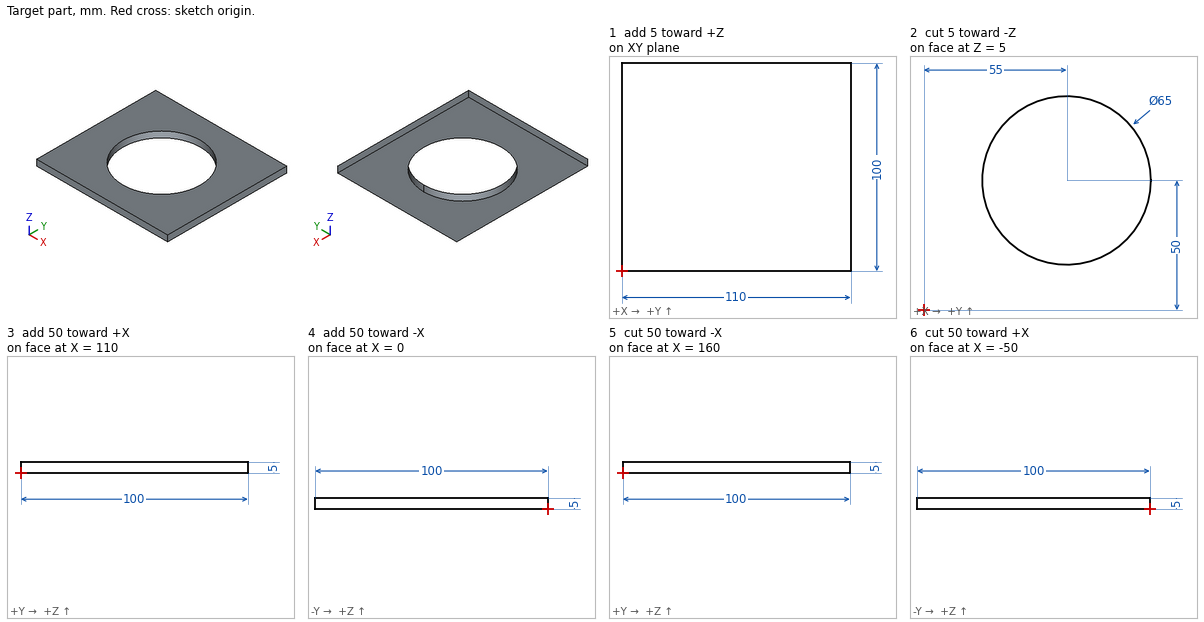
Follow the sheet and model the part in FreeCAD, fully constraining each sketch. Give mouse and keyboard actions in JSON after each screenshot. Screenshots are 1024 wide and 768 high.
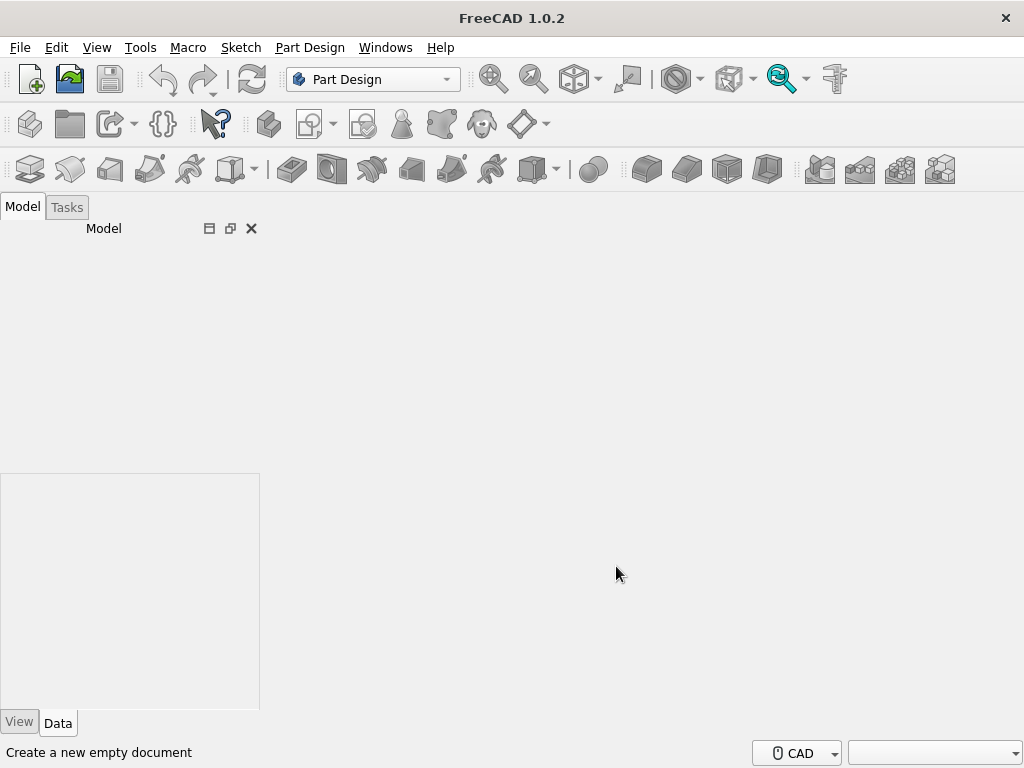
{"action": "left_click", "coordinate": [30, 80]}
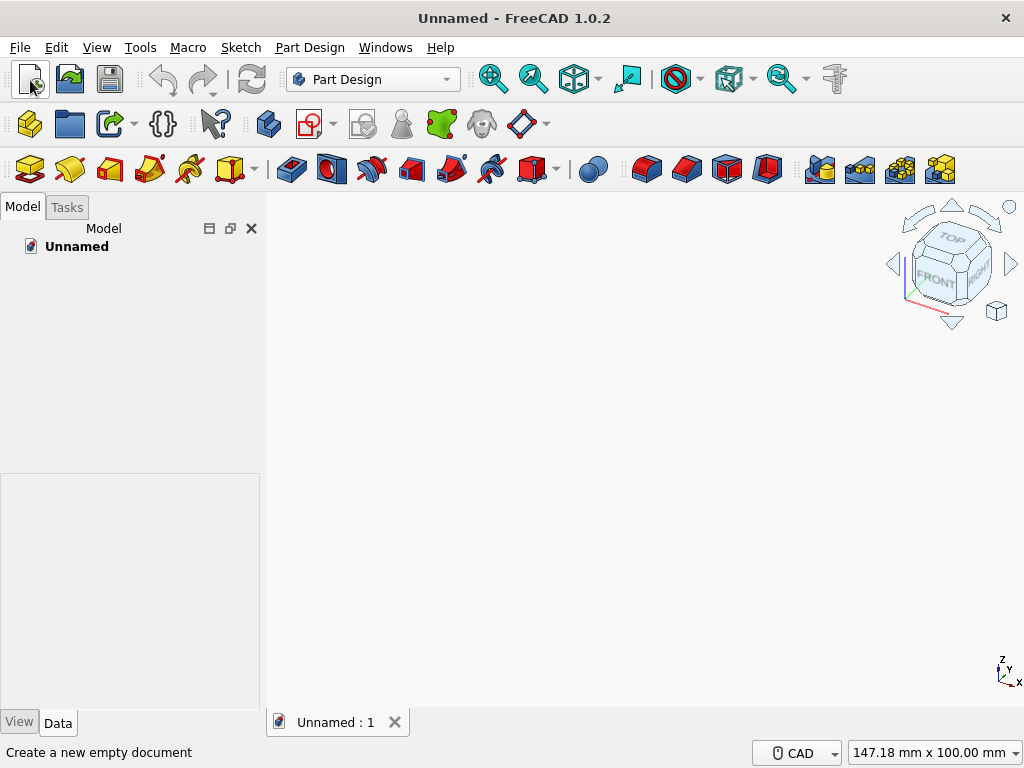
{"action": "left_click", "coordinate": [310, 124]}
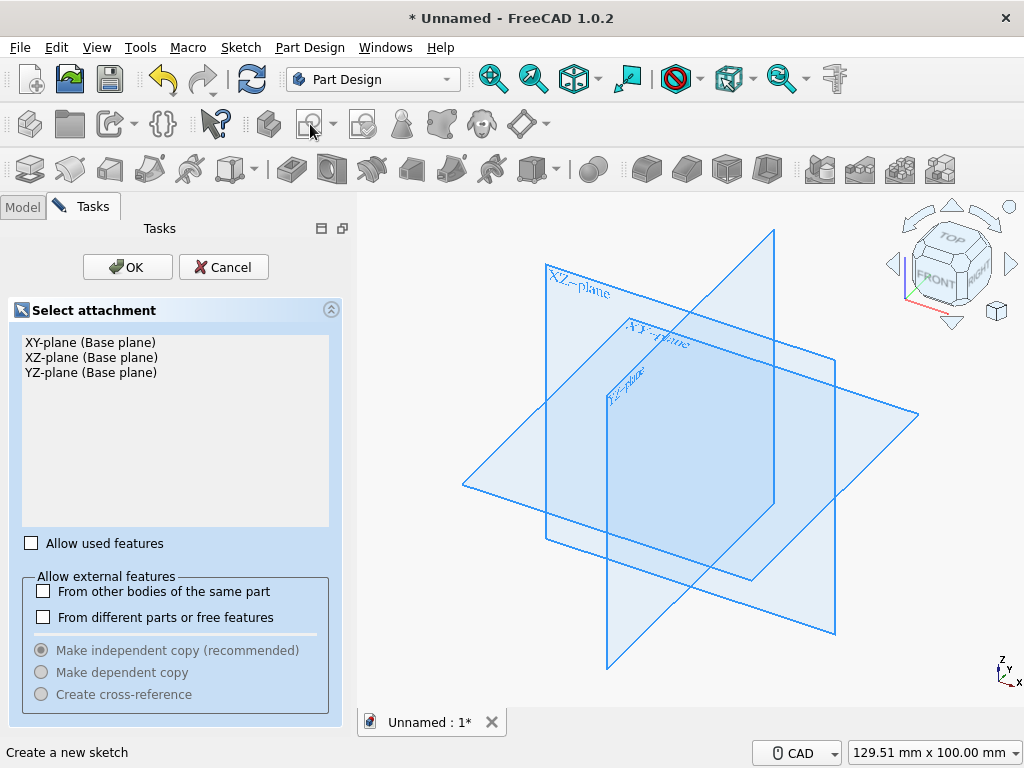
{"action": "left_click", "coordinate": [82, 342]}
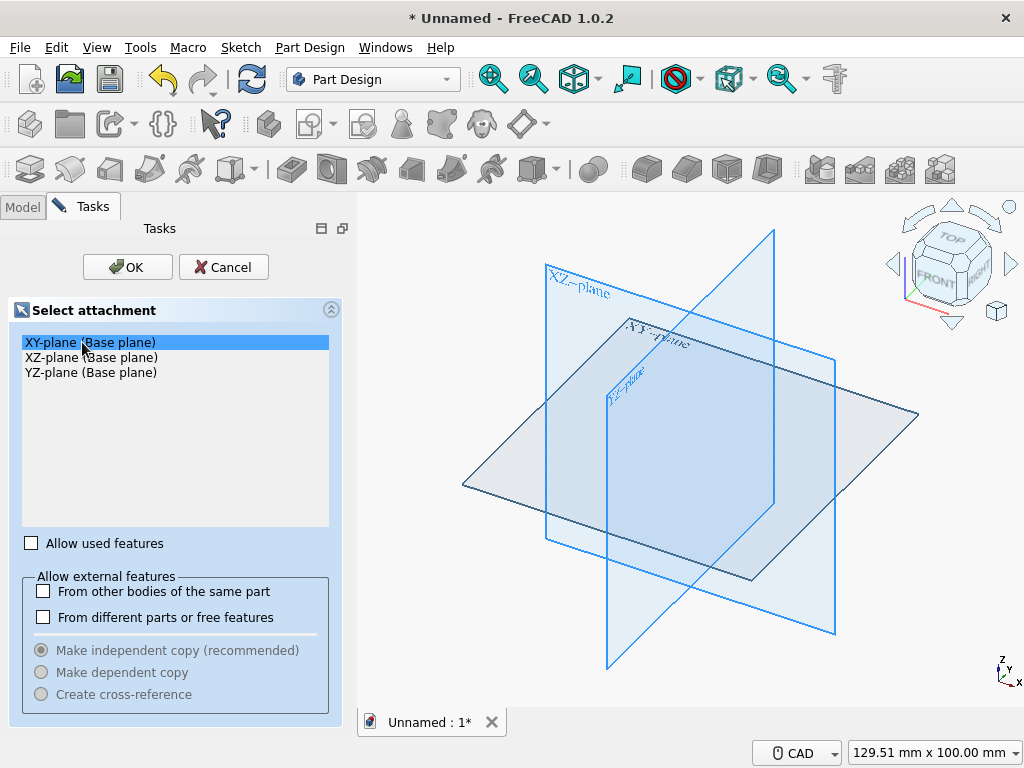
{"action": "left_click", "coordinate": [128, 267]}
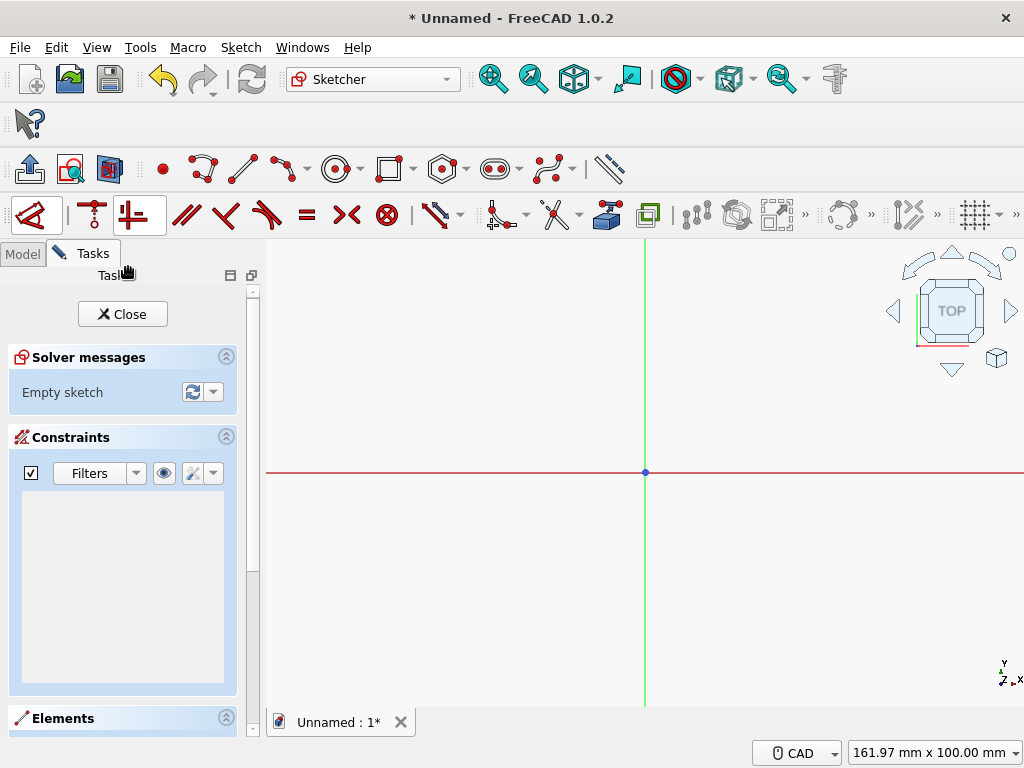
{"action": "scroll", "coordinate": [294, 679], "scroll_direction": "down", "scroll_amount": 3}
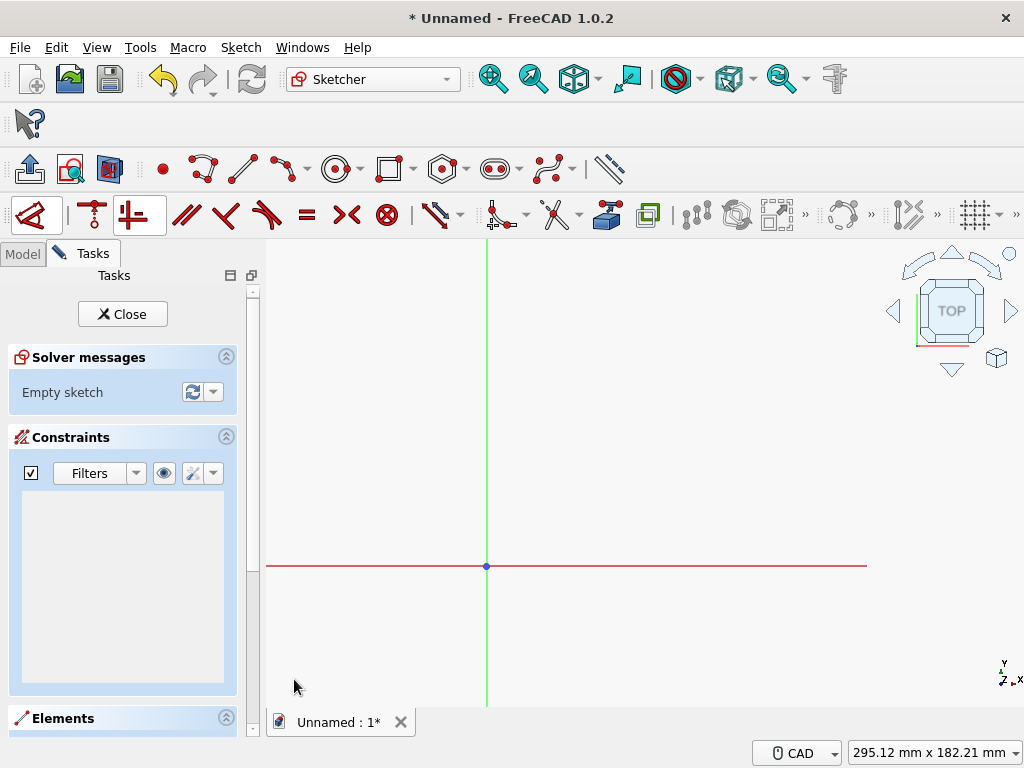
{"action": "left_click", "coordinate": [390, 170]}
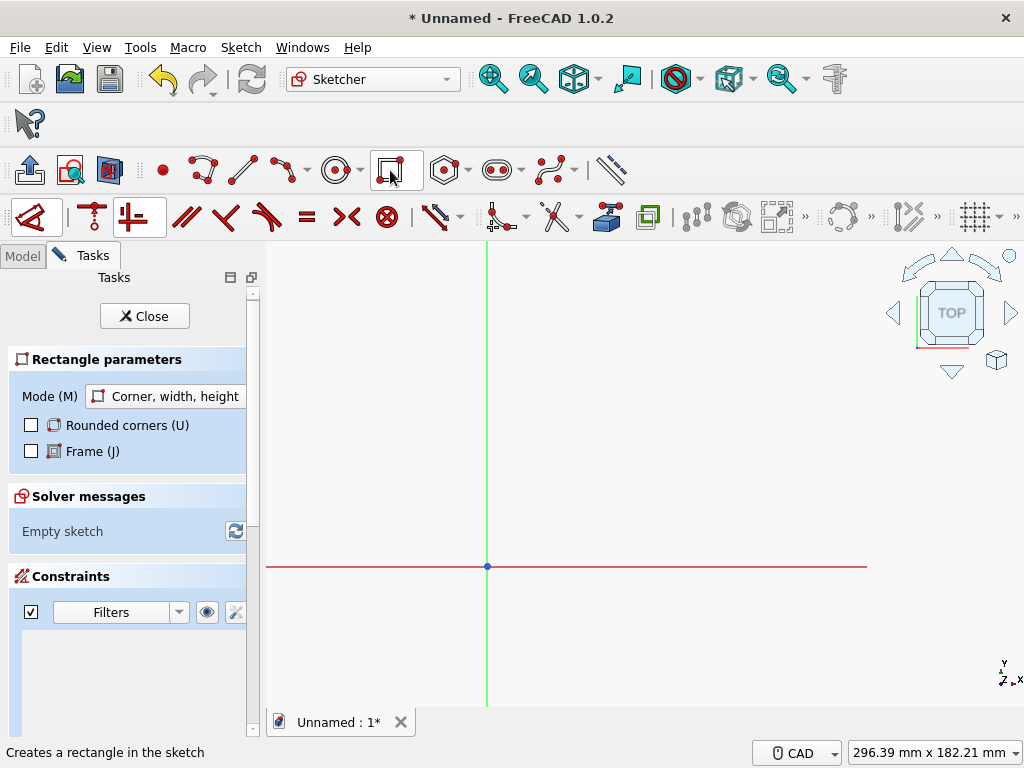
{"action": "left_click", "coordinate": [487, 567]}
{"action": "left_click", "coordinate": [769, 311]}
{"action": "key", "text": "Escape"}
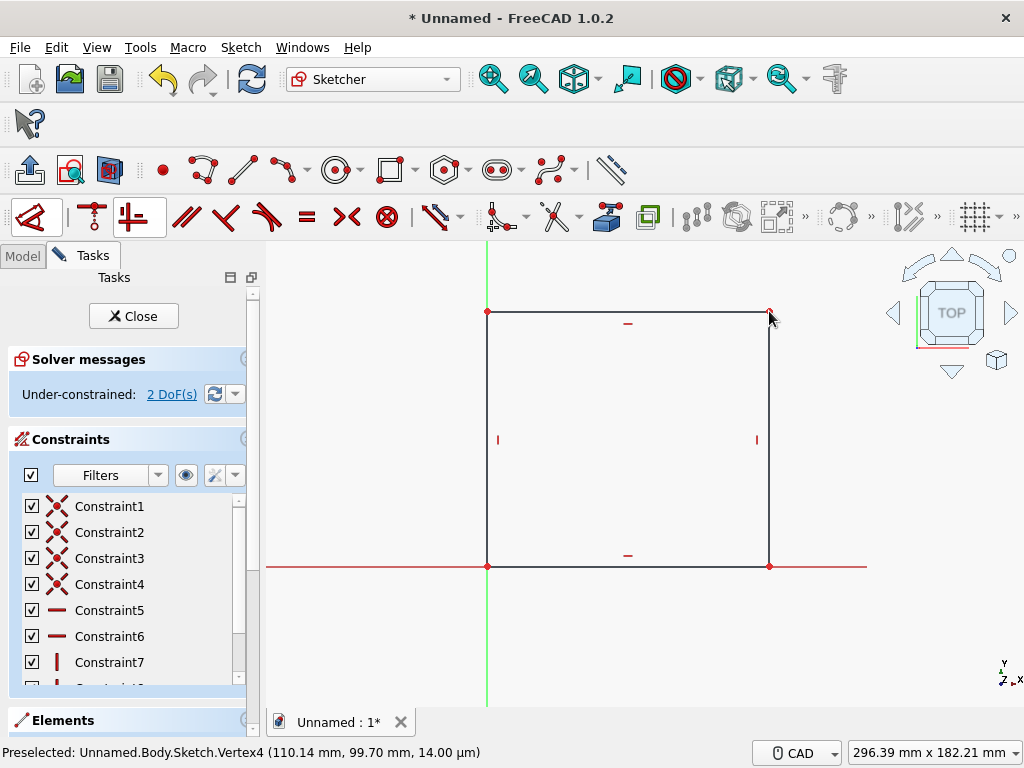
{"action": "left_click", "coordinate": [30, 218]}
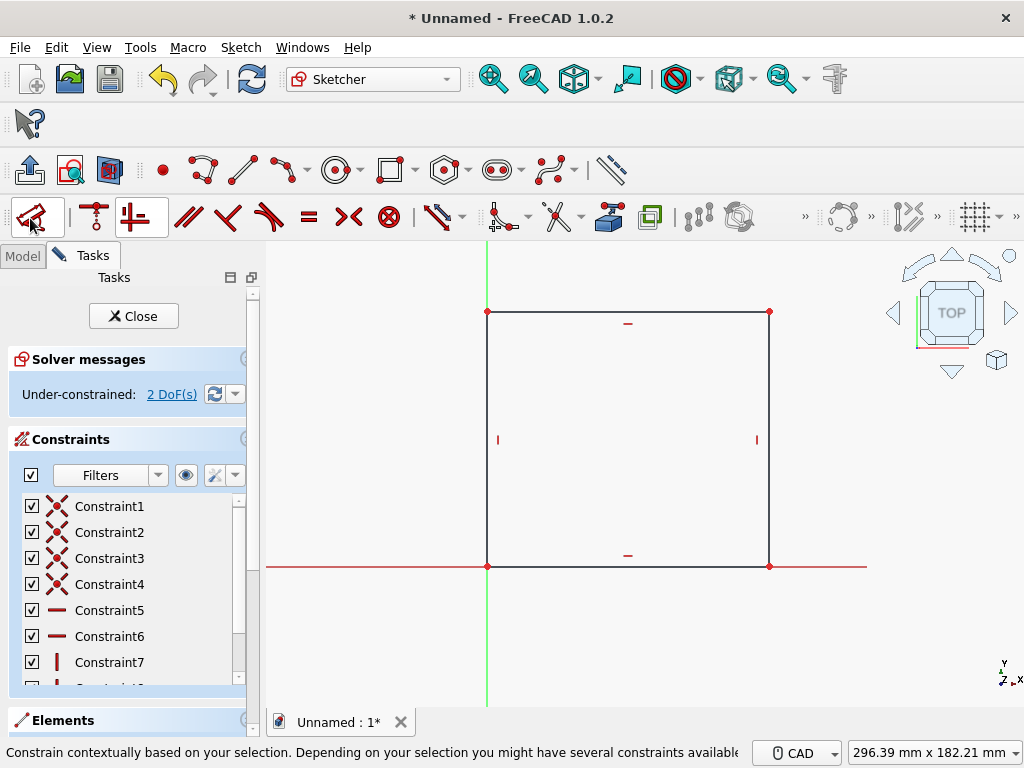
{"action": "left_click", "coordinate": [572, 567]}
{"action": "left_click", "coordinate": [628, 601]}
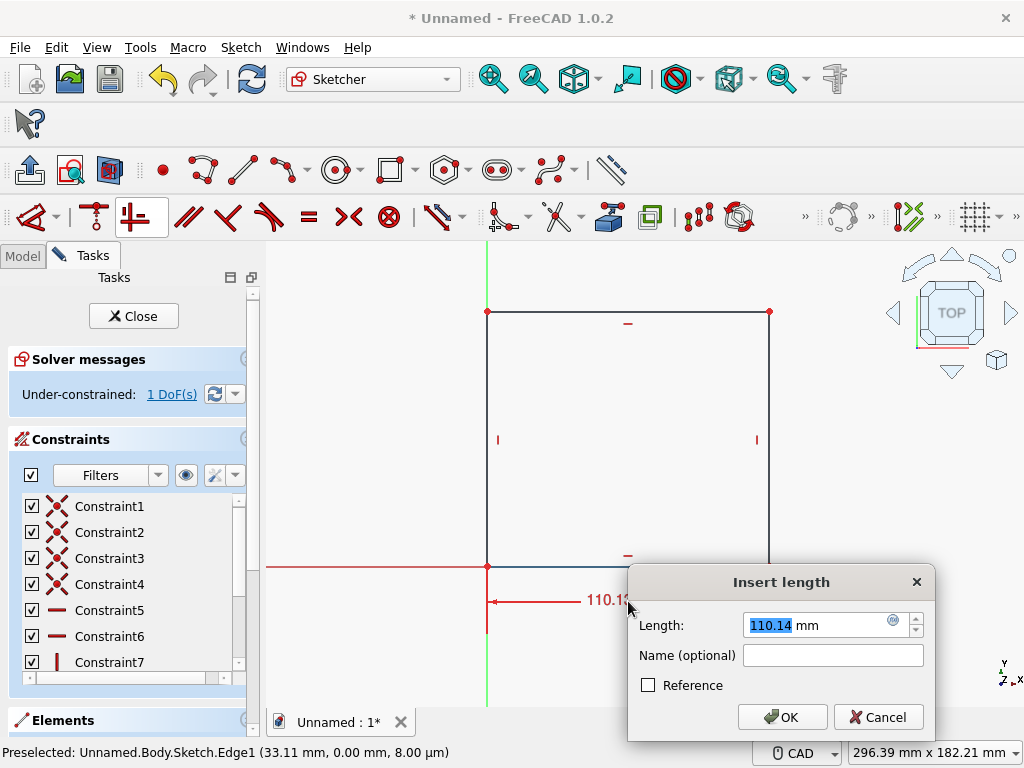
{"action": "type", "text": "110"}
{"action": "key", "text": "Return"}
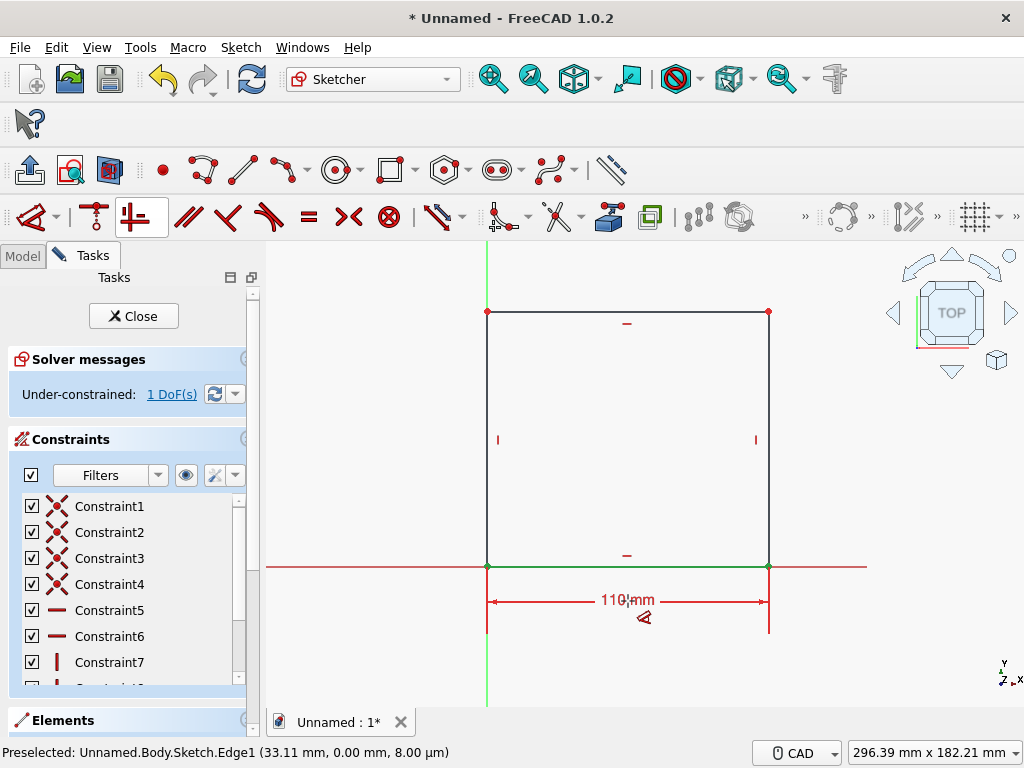
{"action": "left_click", "coordinate": [769, 490]}
{"action": "left_click", "coordinate": [803, 439]}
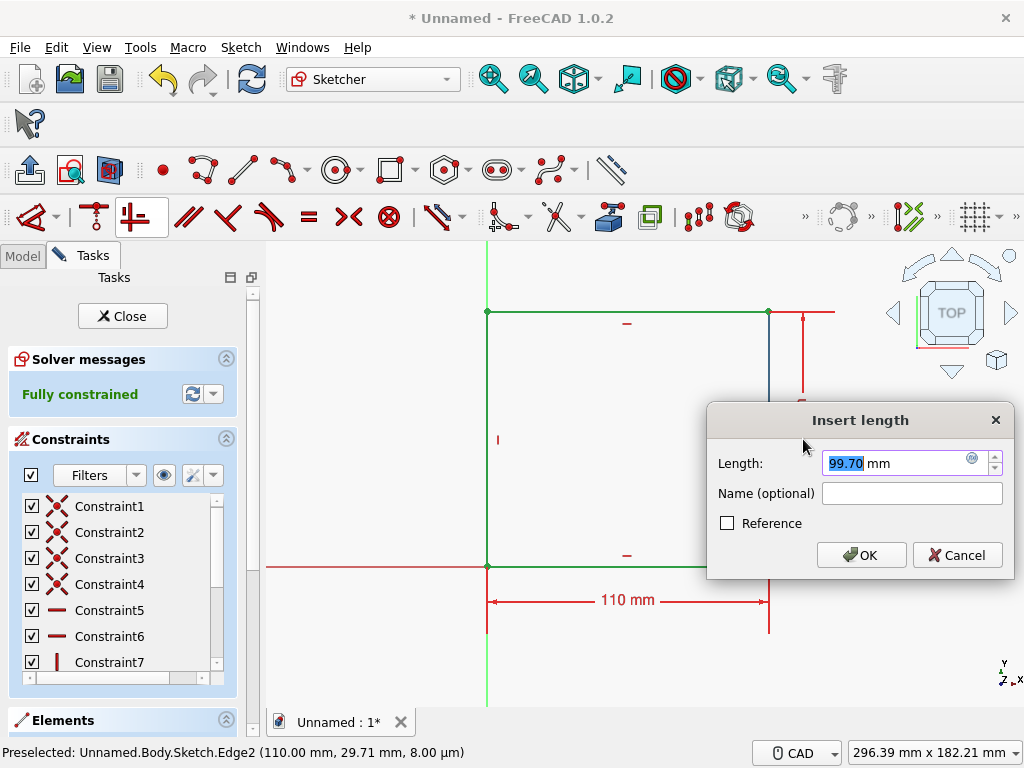
{"action": "type", "text": "100"}
{"action": "key", "text": "Return"}
{"action": "key", "text": "Escape"}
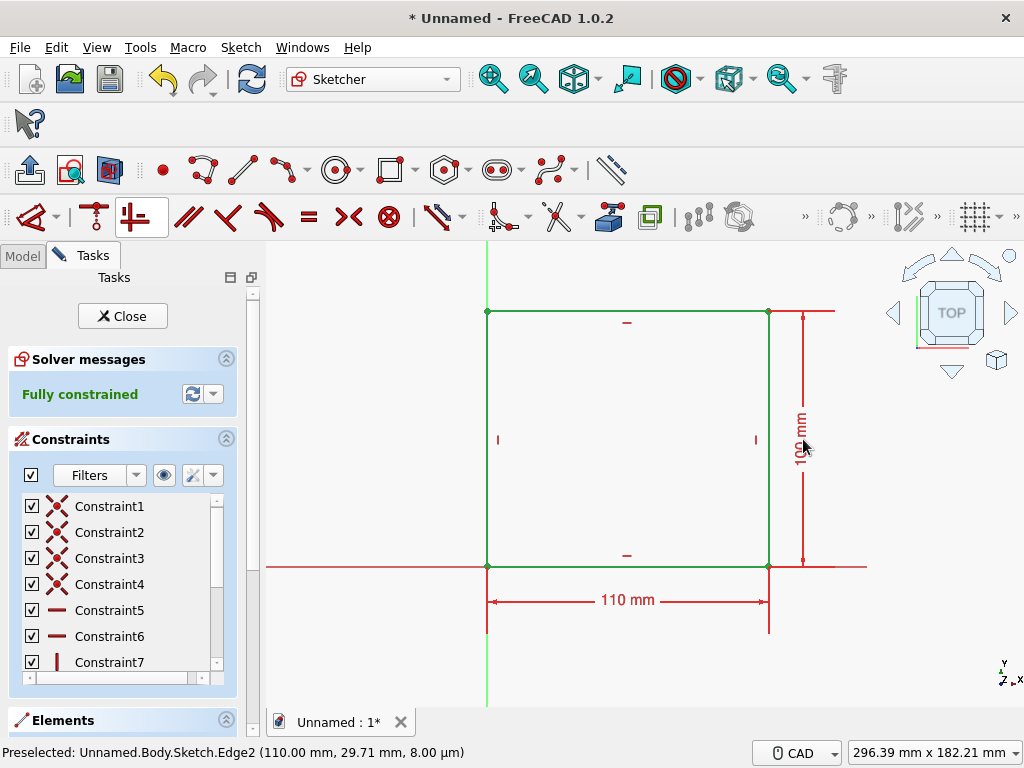
{"action": "left_click", "coordinate": [123, 316]}